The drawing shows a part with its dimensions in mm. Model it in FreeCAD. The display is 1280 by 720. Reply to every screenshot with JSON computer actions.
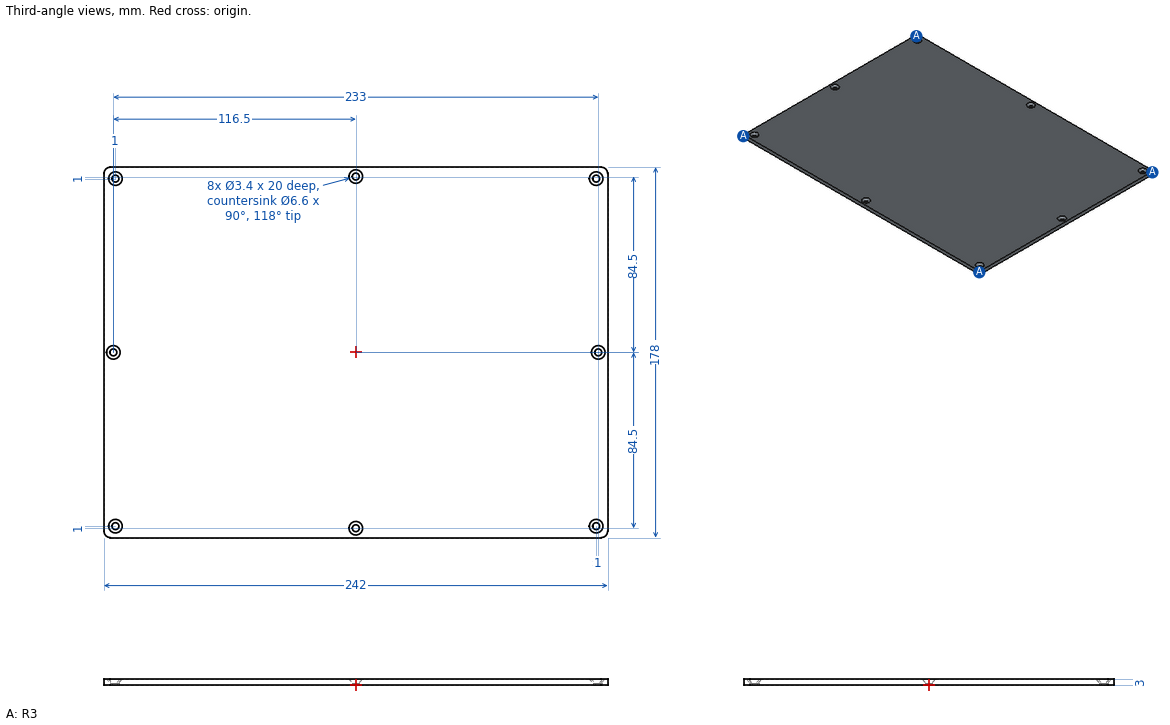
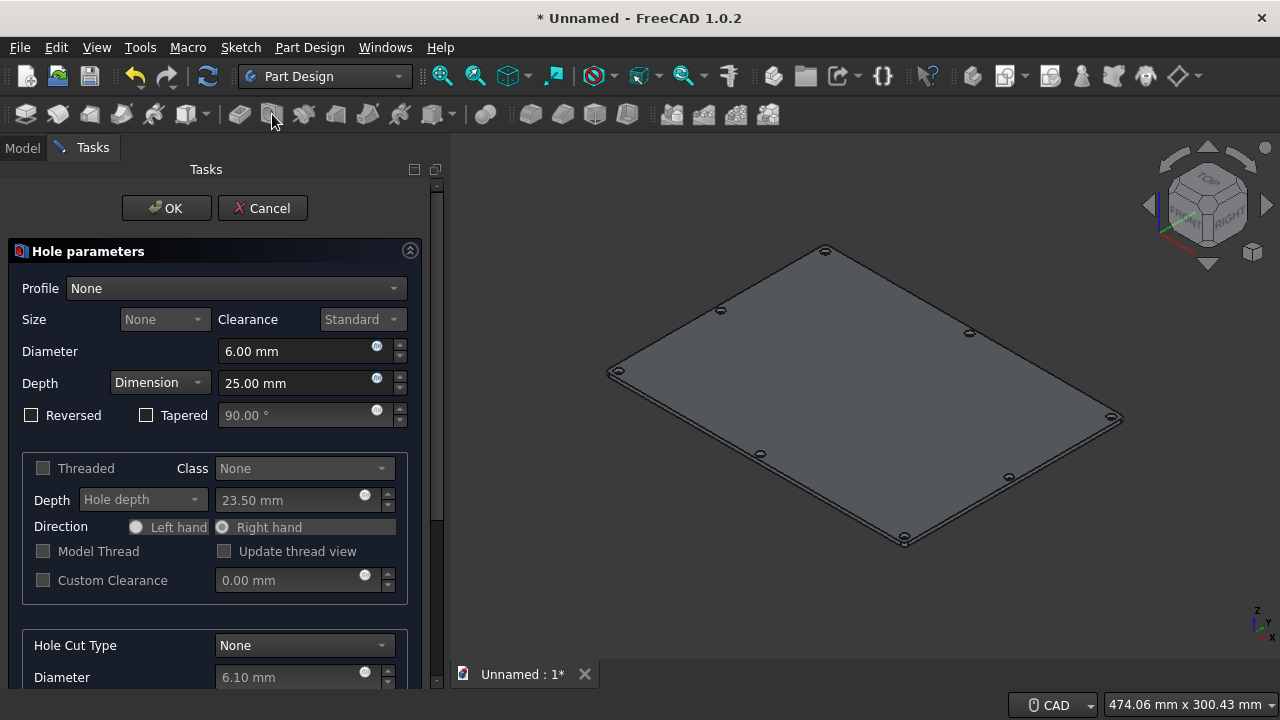
{"action": "triple_click", "coordinate": [305, 351]}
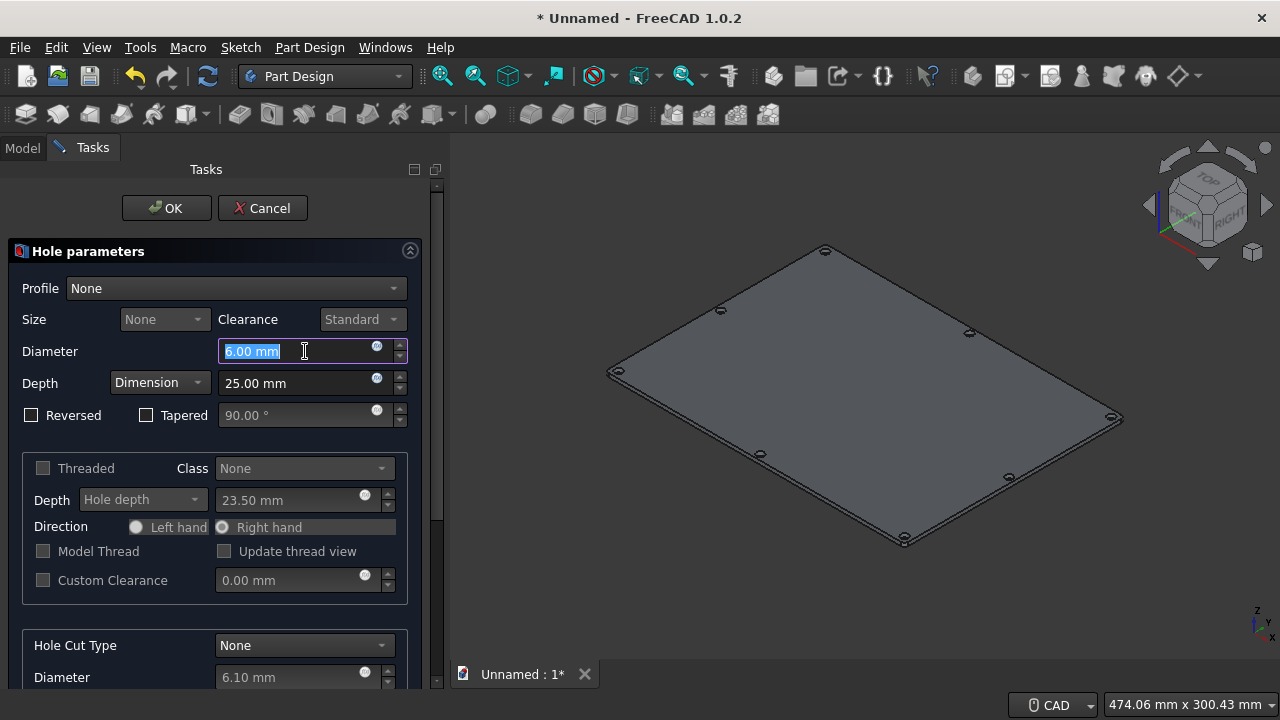
{"action": "type", "text": "3.4"}
{"action": "key", "text": "Tab"}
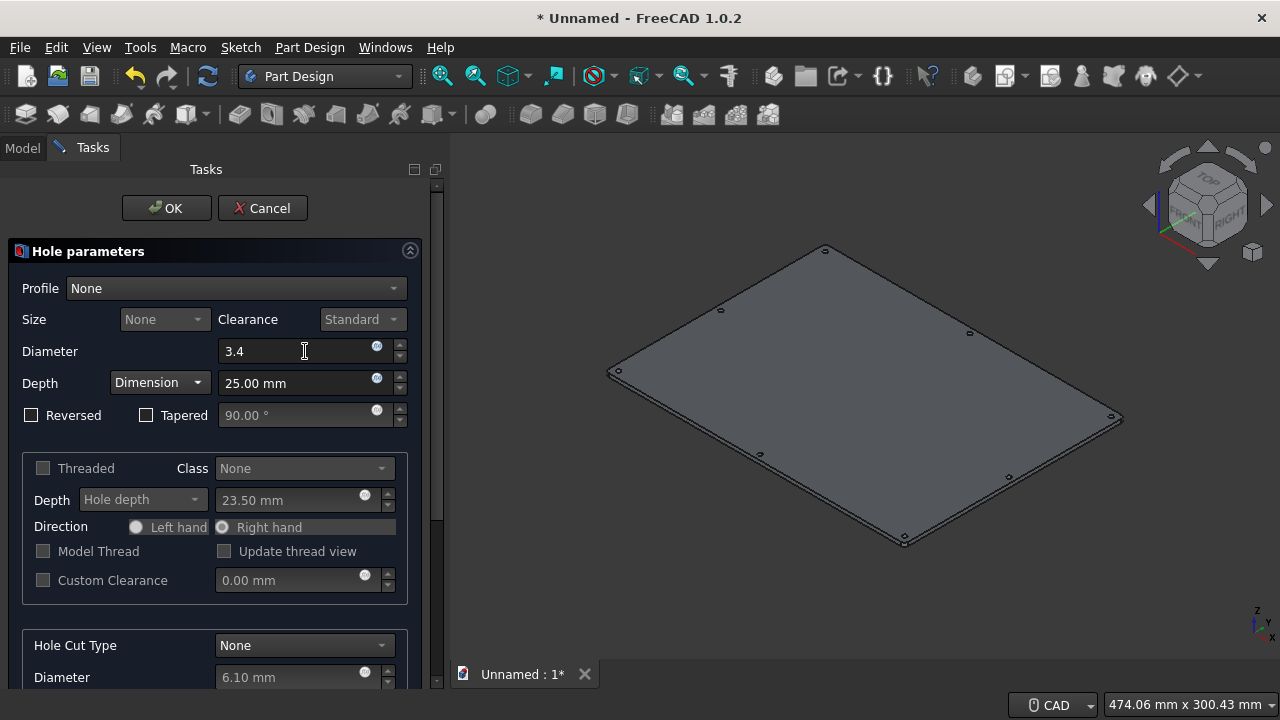
{"action": "triple_click", "coordinate": [305, 383]}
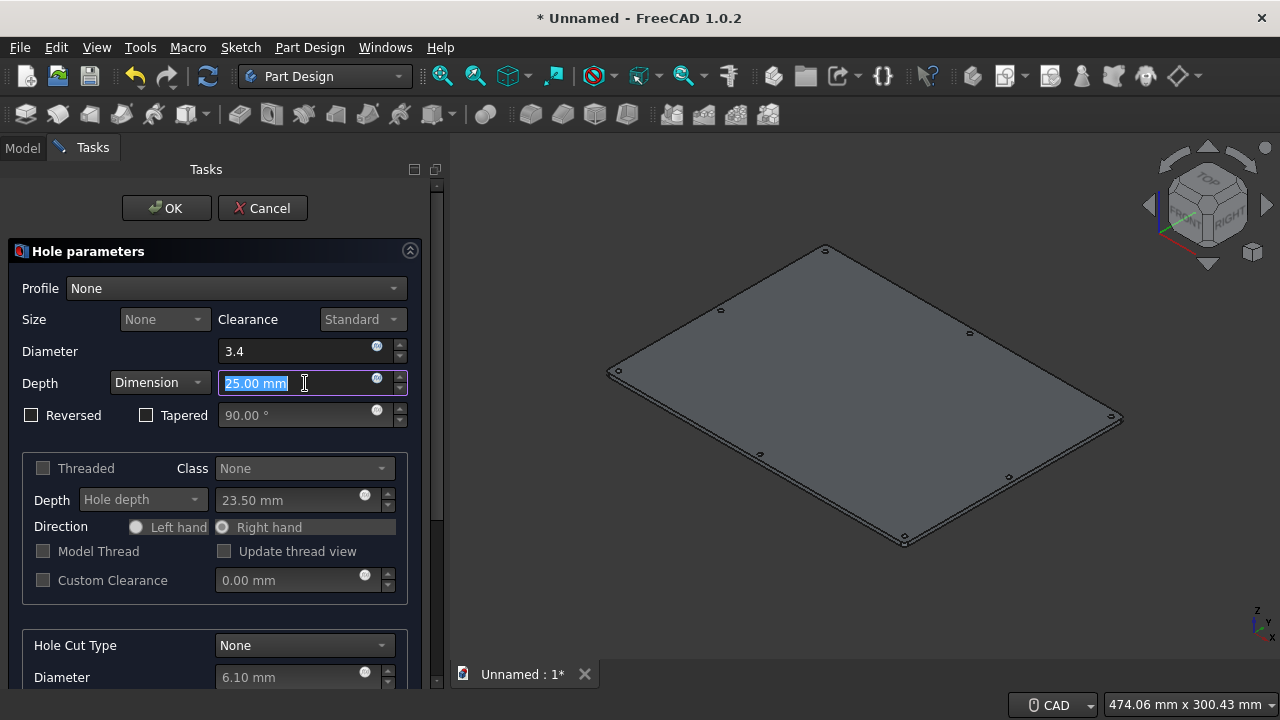
{"action": "type", "text": "20"}
{"action": "key", "text": "Tab"}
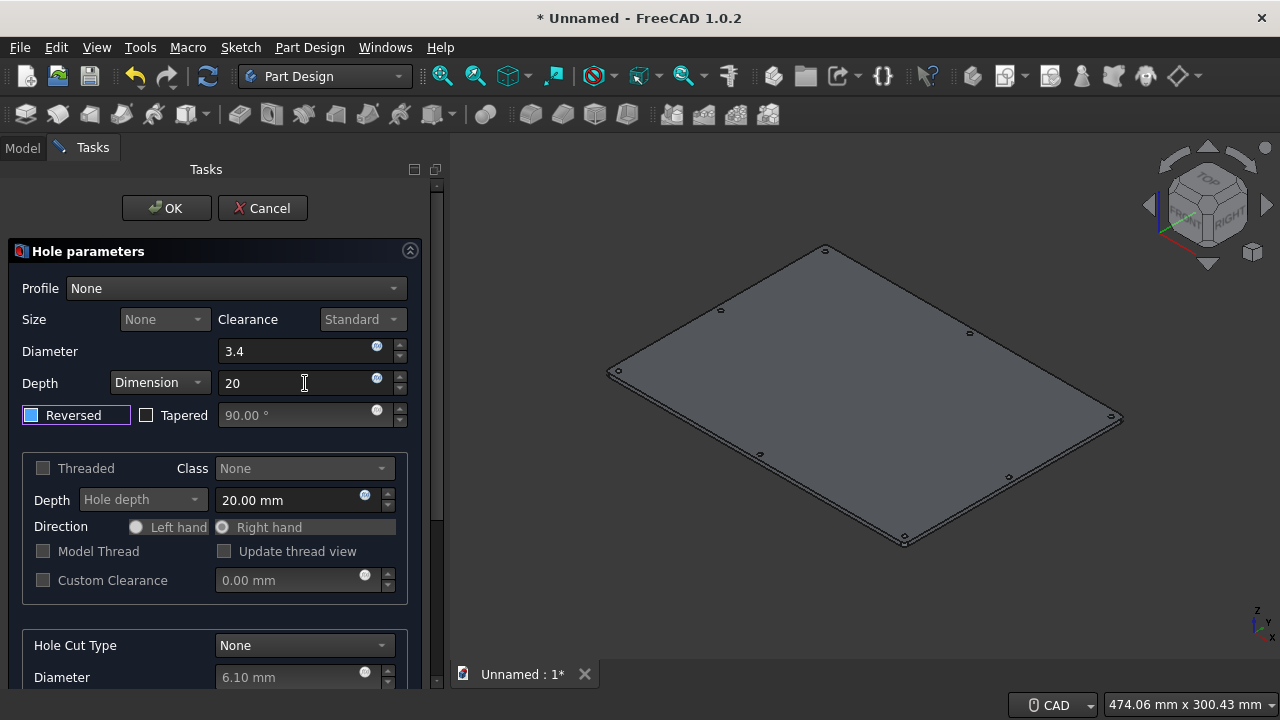
{"action": "left_click", "coordinate": [306, 646]}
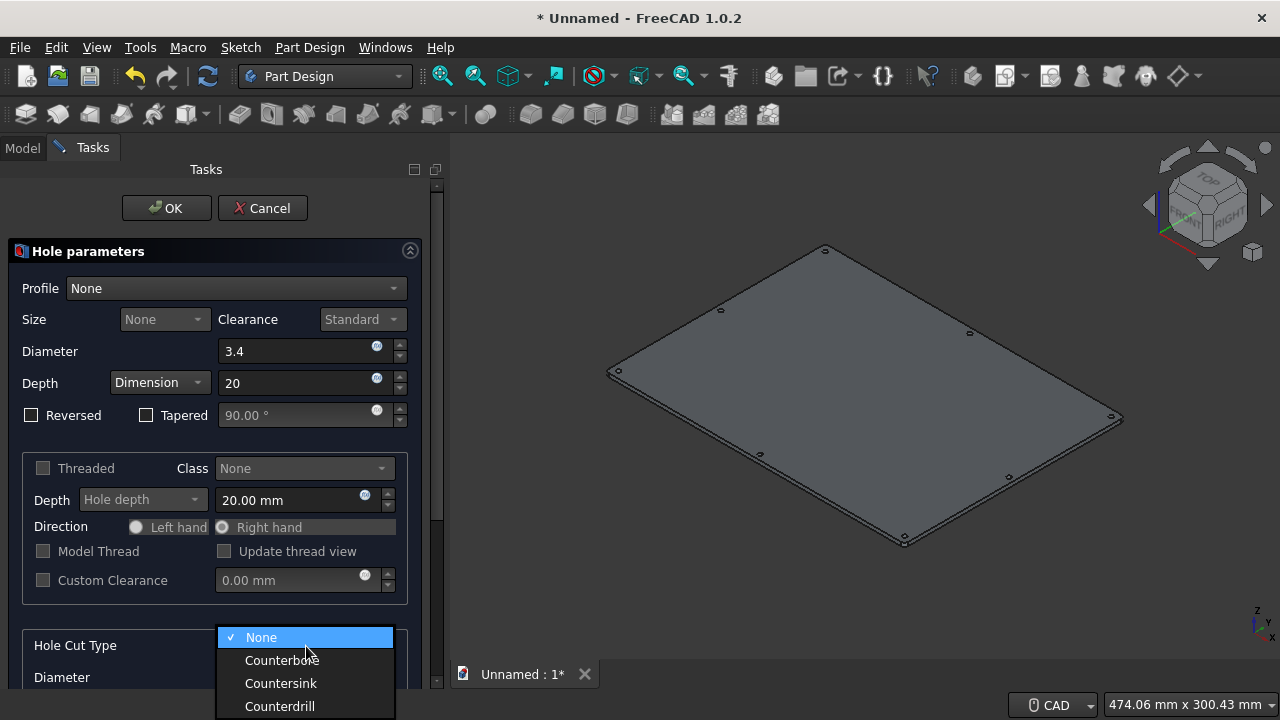
{"action": "left_click", "coordinate": [304, 684]}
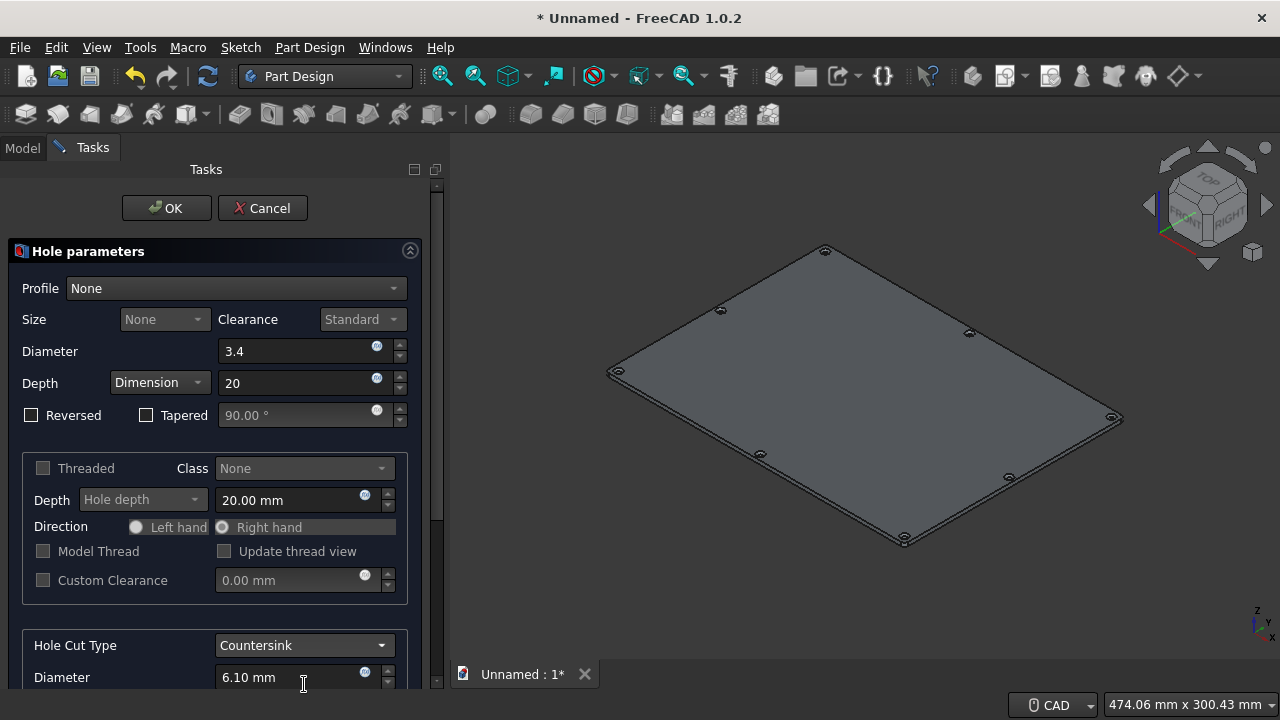
{"action": "scroll", "coordinate": [437, 434], "scroll_direction": "down", "scroll_amount": 2}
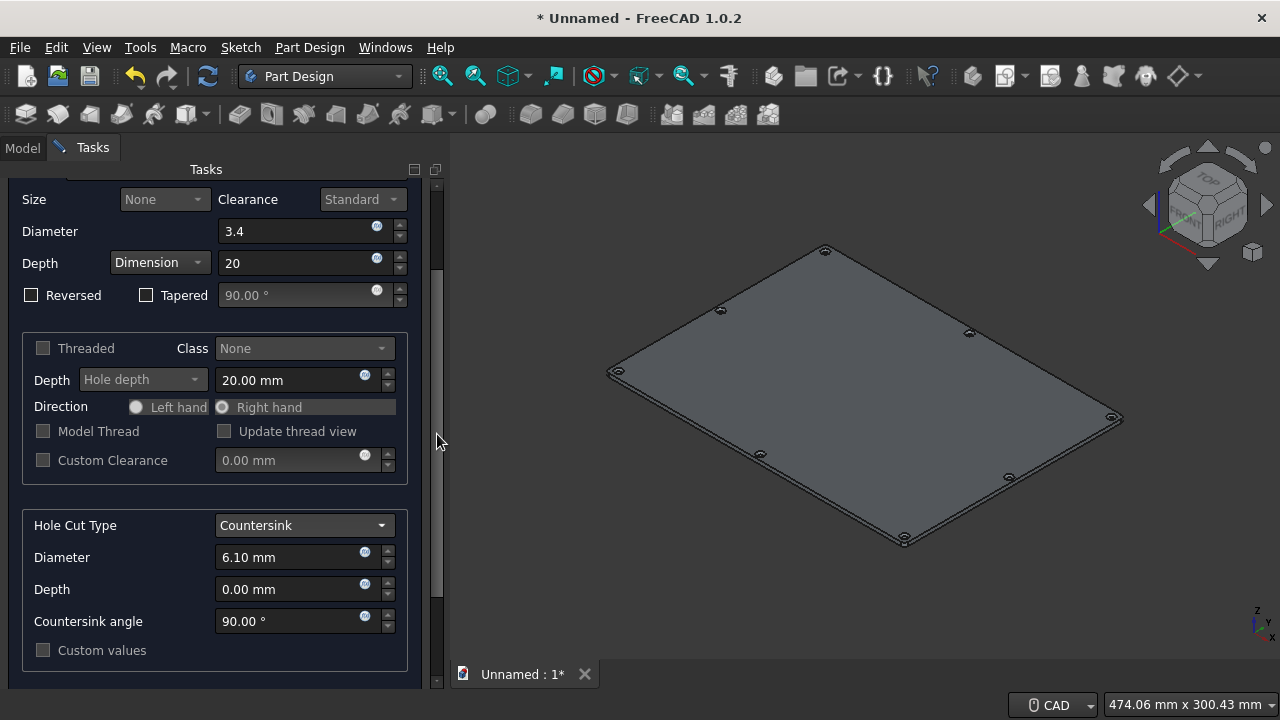
{"action": "triple_click", "coordinate": [298, 557]}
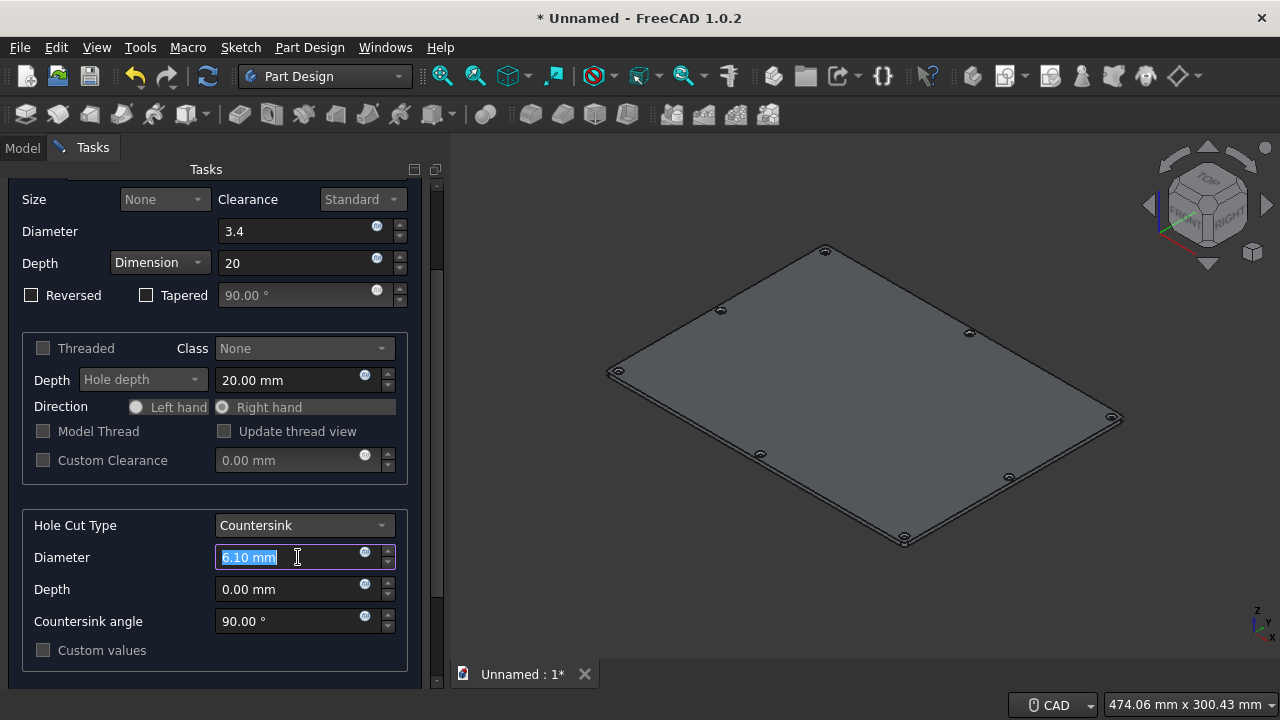
{"action": "type", "text": "6.6"}
{"action": "key", "text": "Tab"}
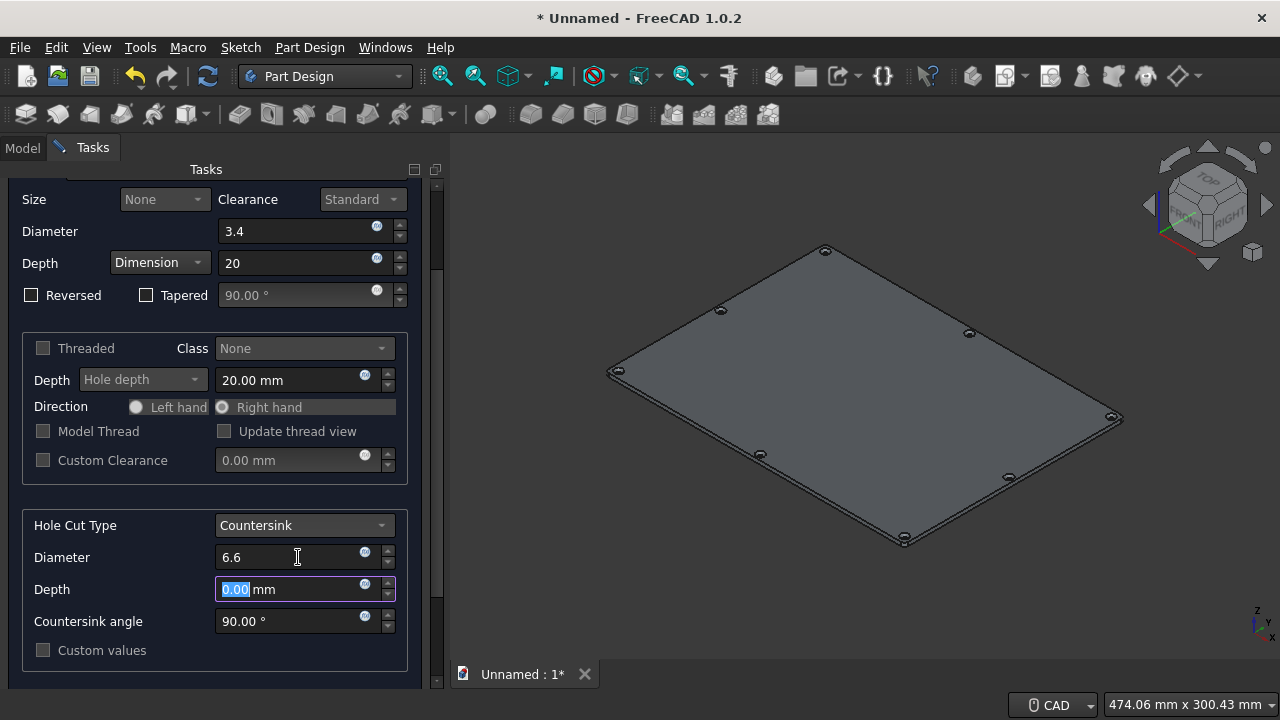
{"action": "scroll", "coordinate": [437, 434], "scroll_direction": "up", "scroll_amount": 3}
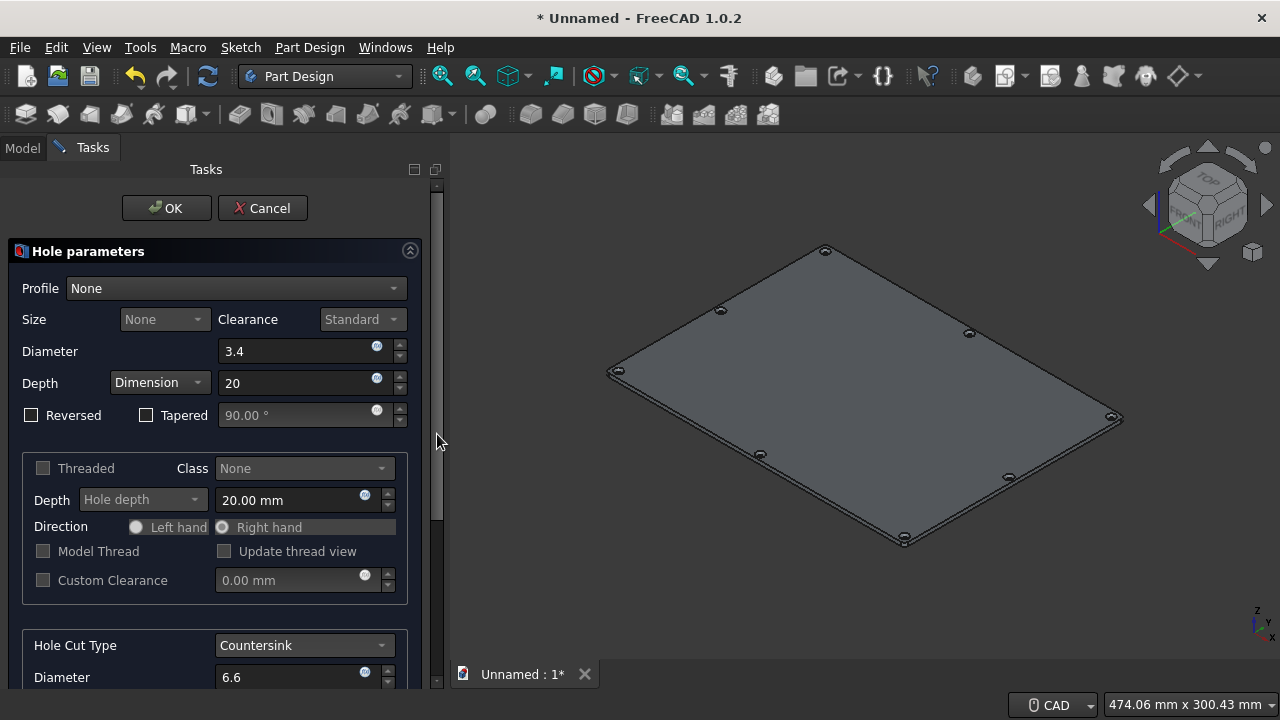
{"action": "left_click", "coordinate": [167, 208]}